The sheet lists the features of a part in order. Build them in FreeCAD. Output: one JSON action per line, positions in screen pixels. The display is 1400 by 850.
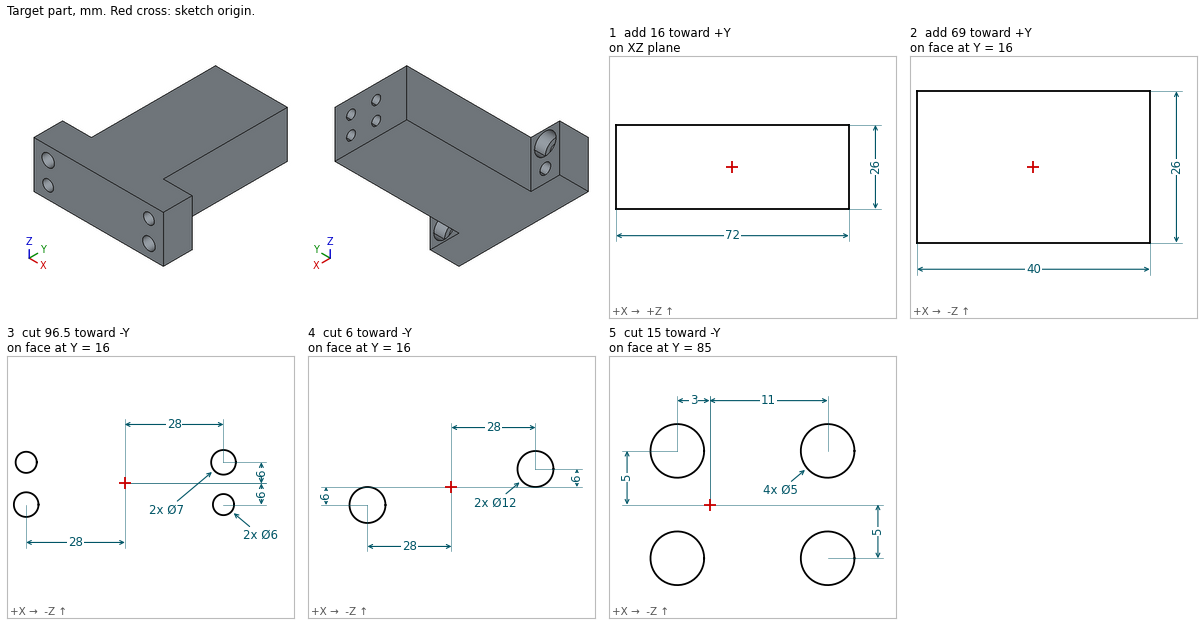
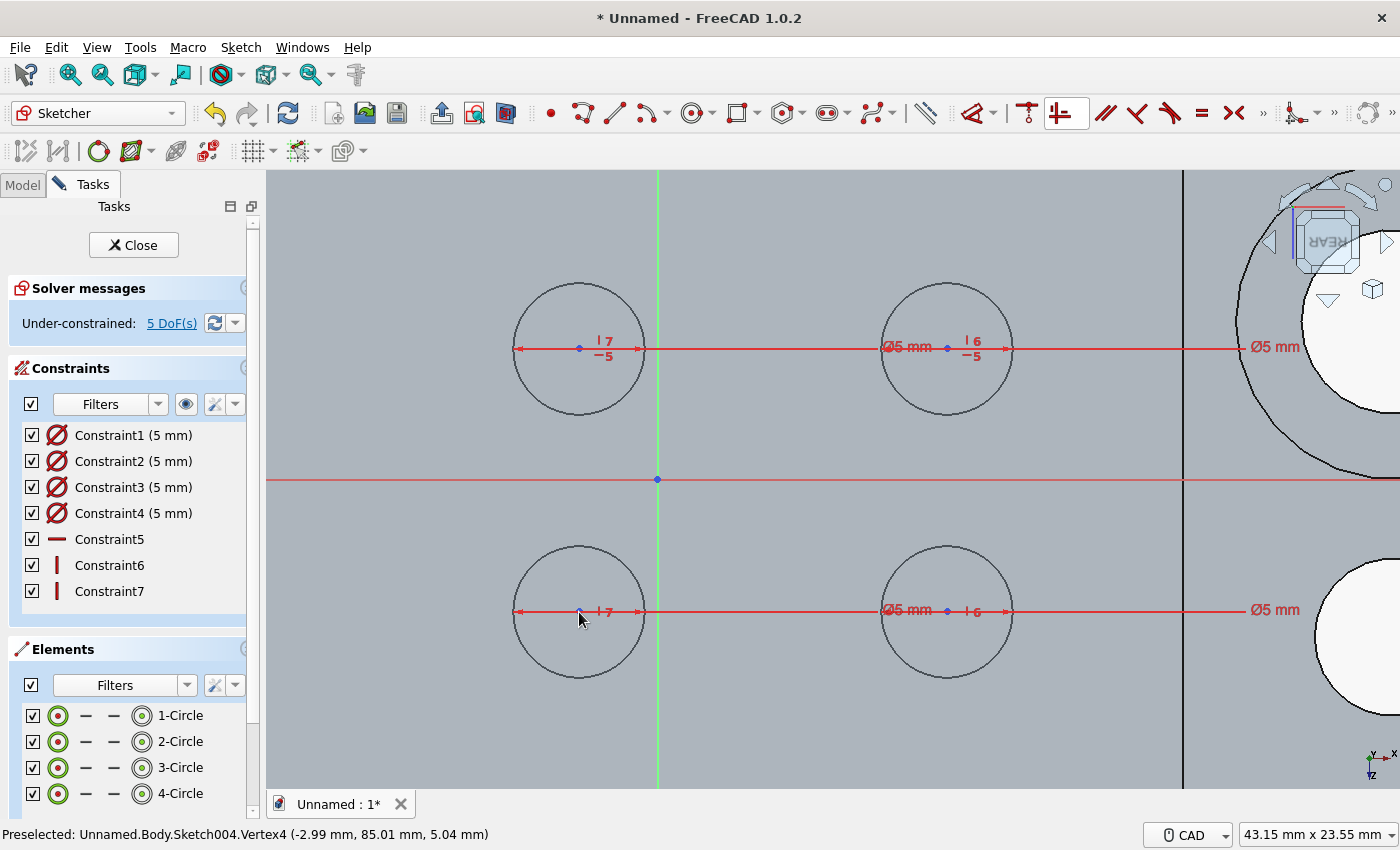
{"action": "left_click", "coordinate": [947, 612]}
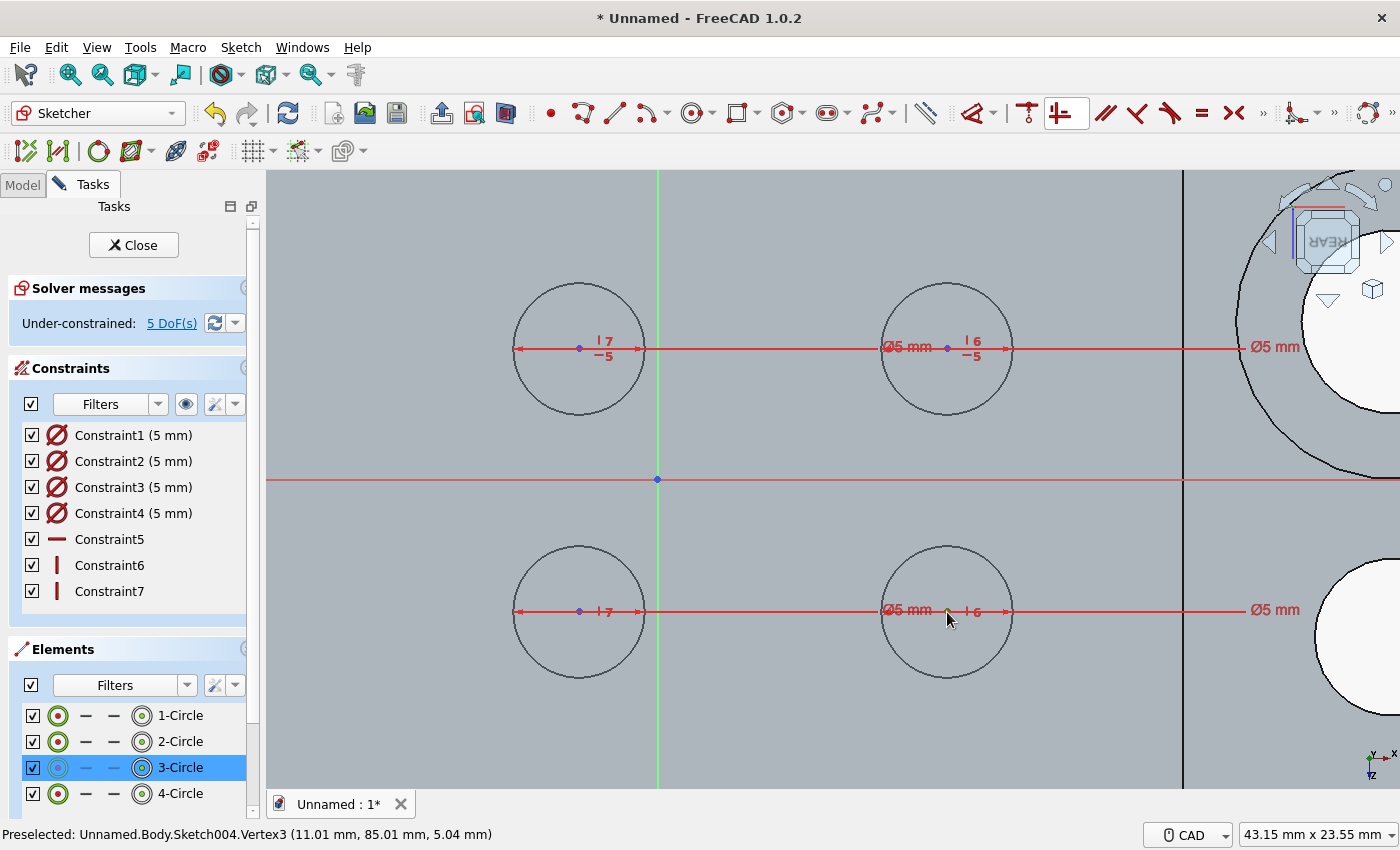
{"action": "left_click", "coordinate": [579, 612]}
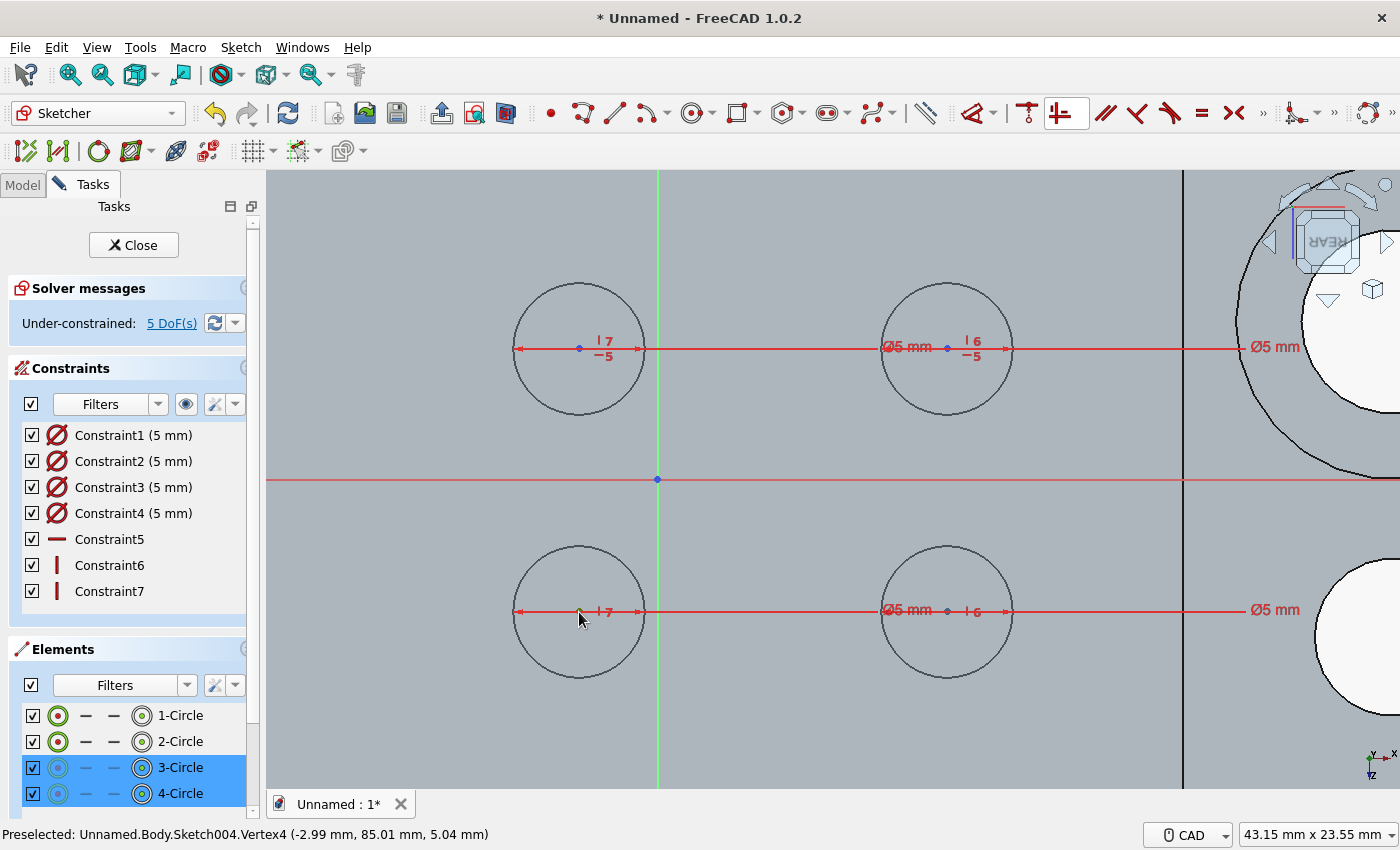
{"action": "key", "text": "h"}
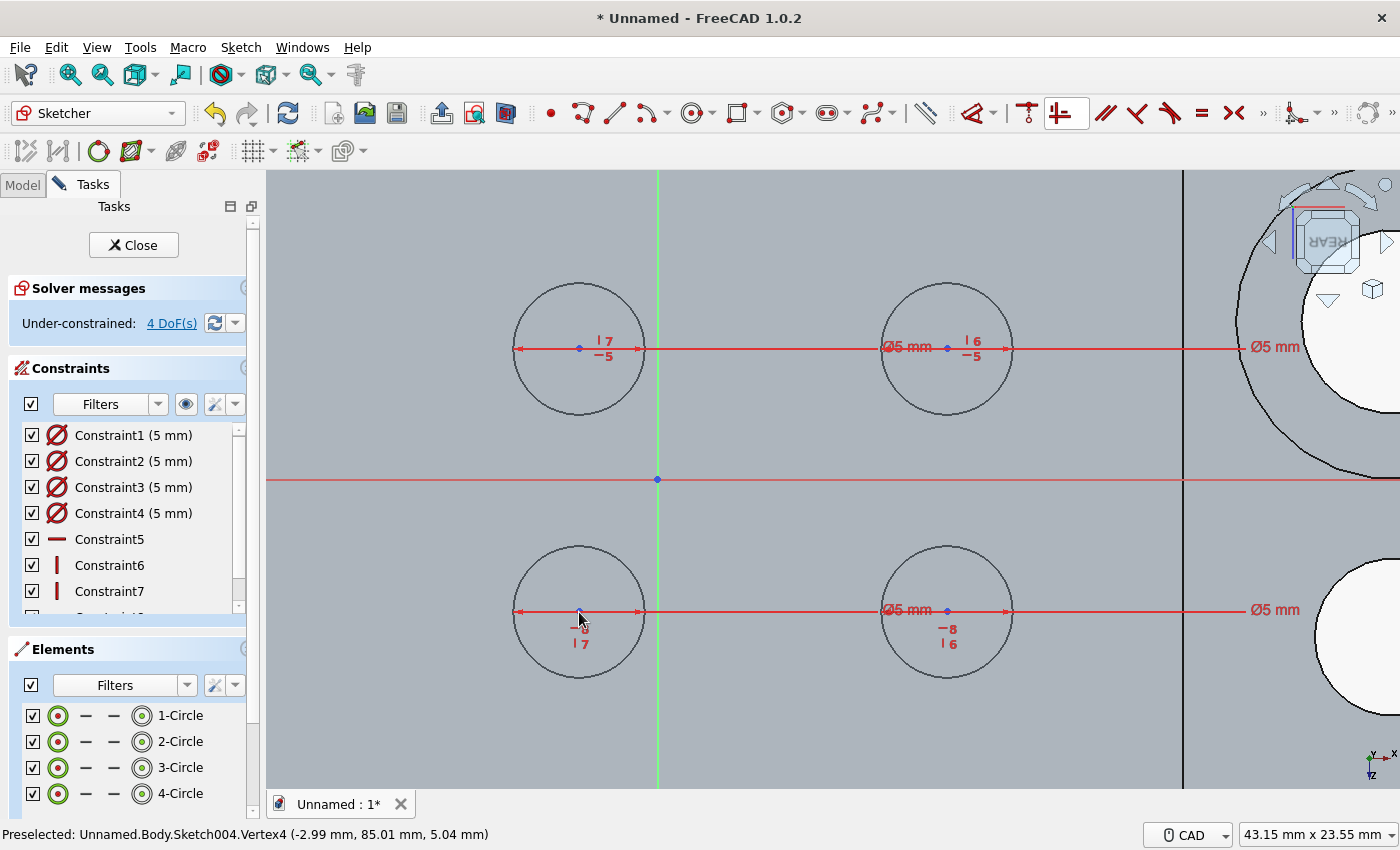
{"action": "left_click", "coordinate": [972, 114]}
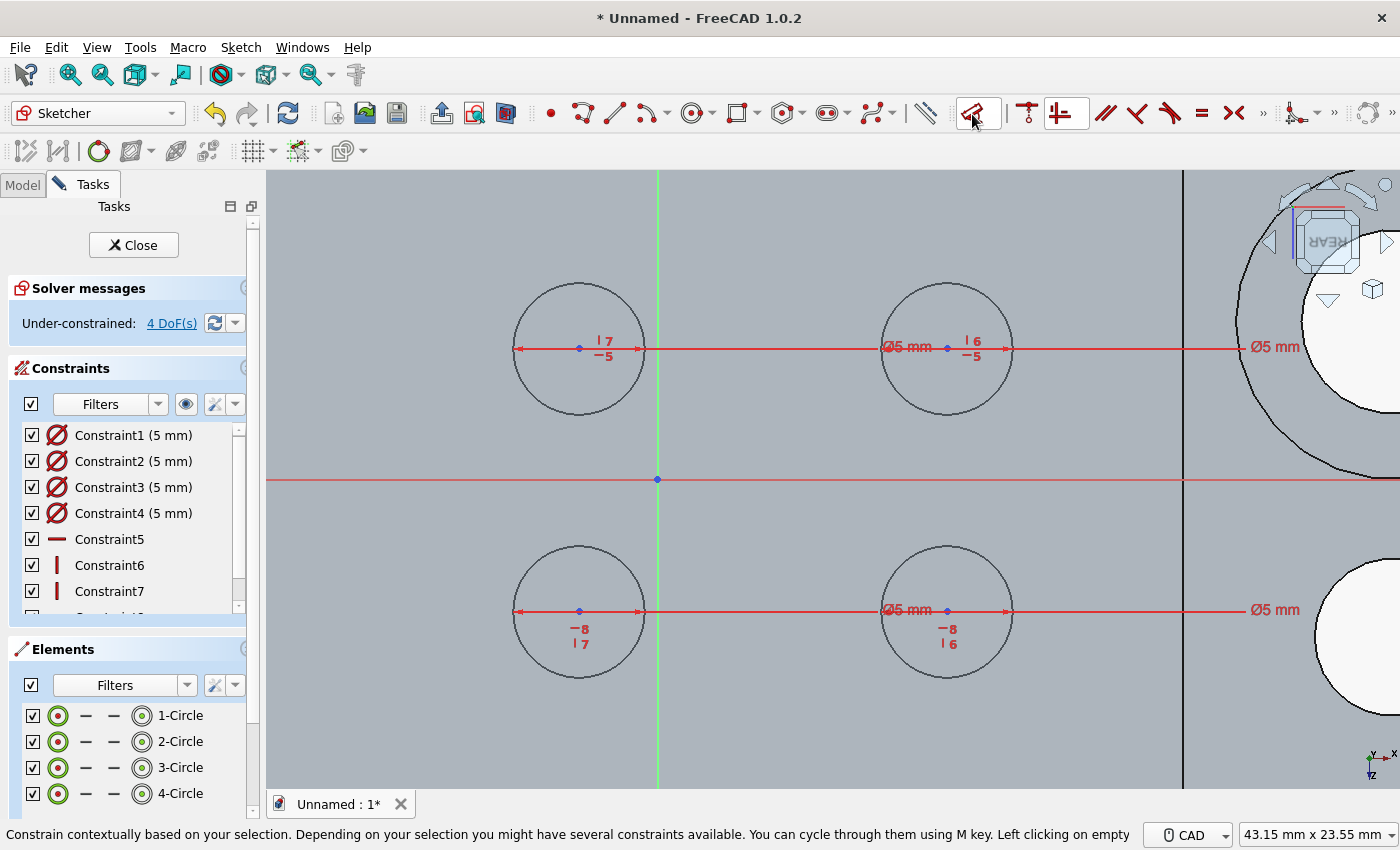
{"action": "left_click", "coordinate": [579, 349]}
{"action": "left_click", "coordinate": [618, 315]}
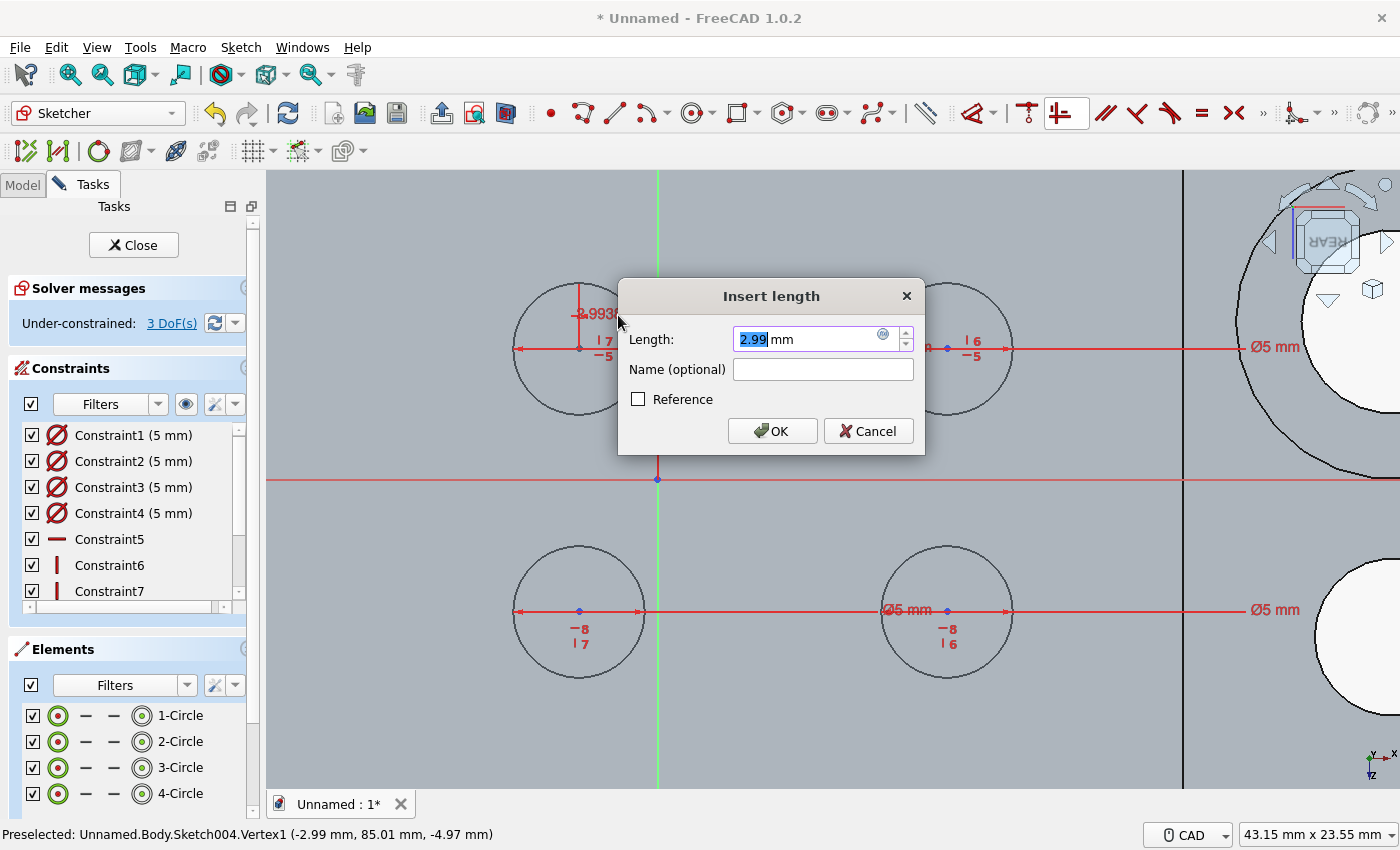
{"action": "type", "text": "3"}
{"action": "key", "text": "Return"}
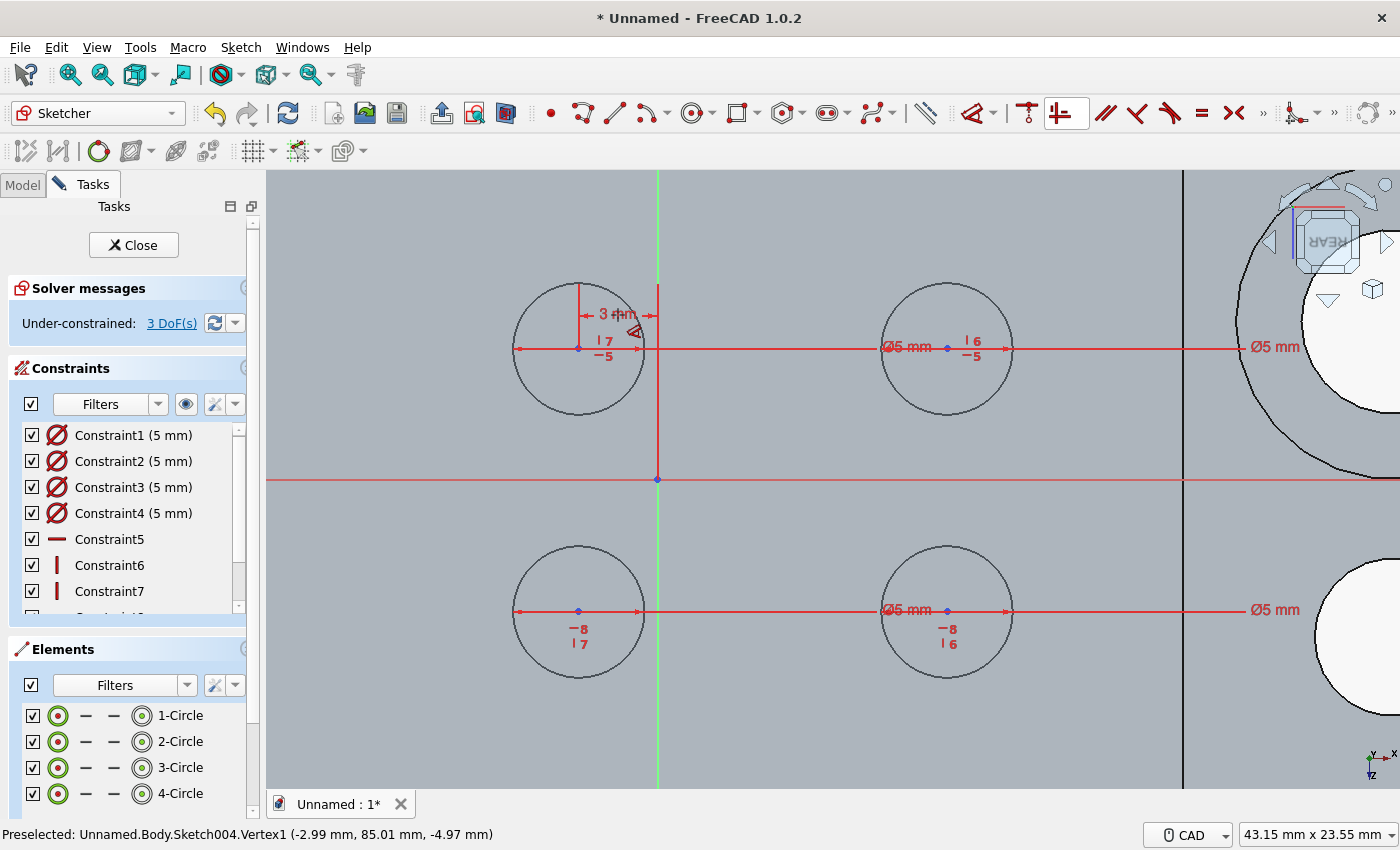
{"action": "left_click", "coordinate": [579, 349]}
{"action": "left_click", "coordinate": [545, 384]}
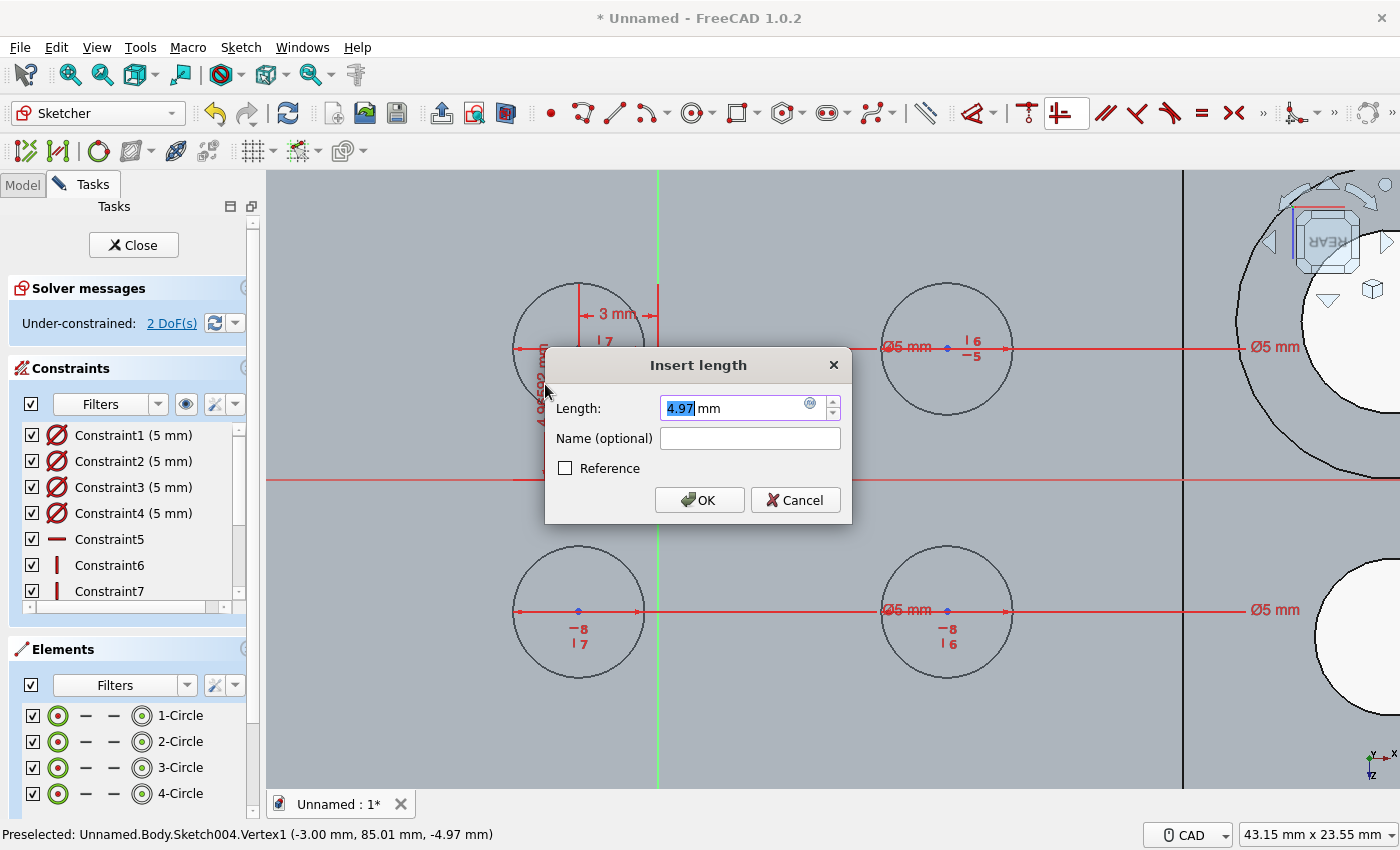
{"action": "type", "text": "5"}
{"action": "key", "text": "Return"}